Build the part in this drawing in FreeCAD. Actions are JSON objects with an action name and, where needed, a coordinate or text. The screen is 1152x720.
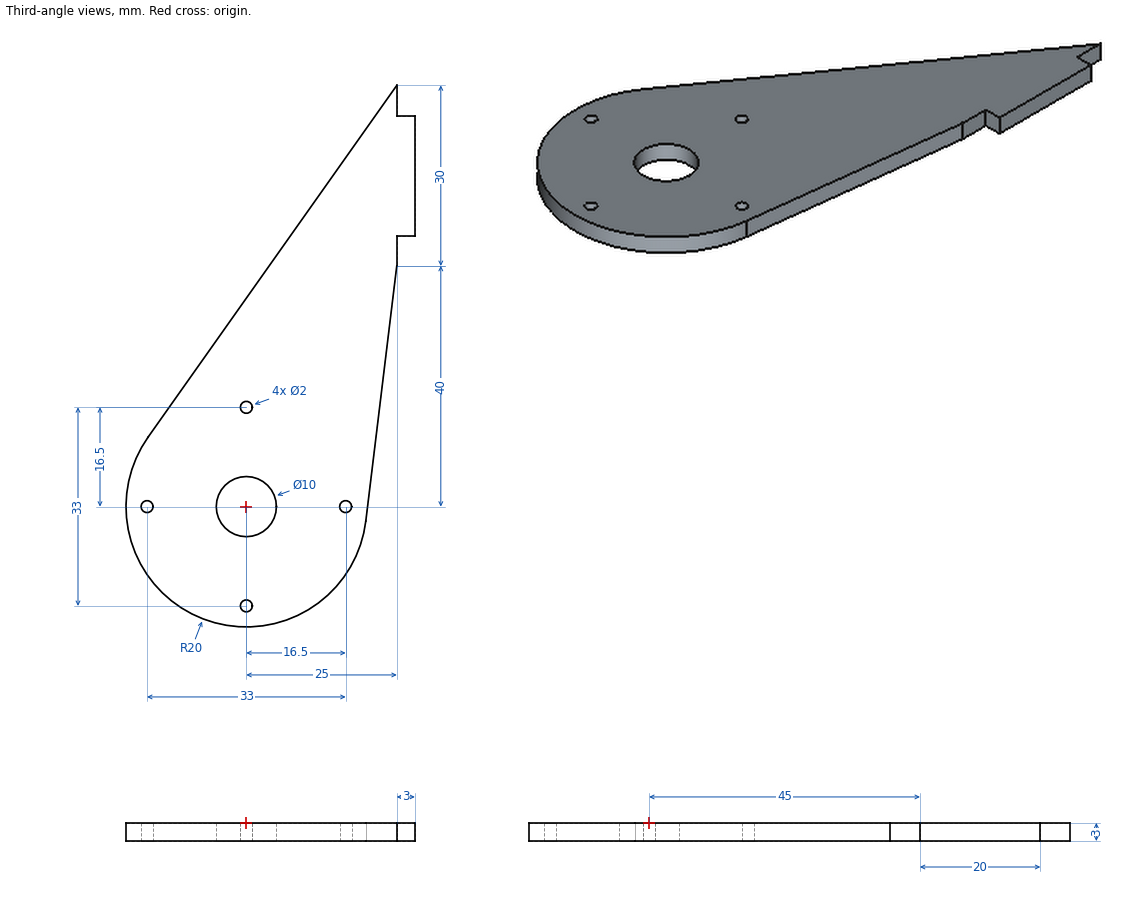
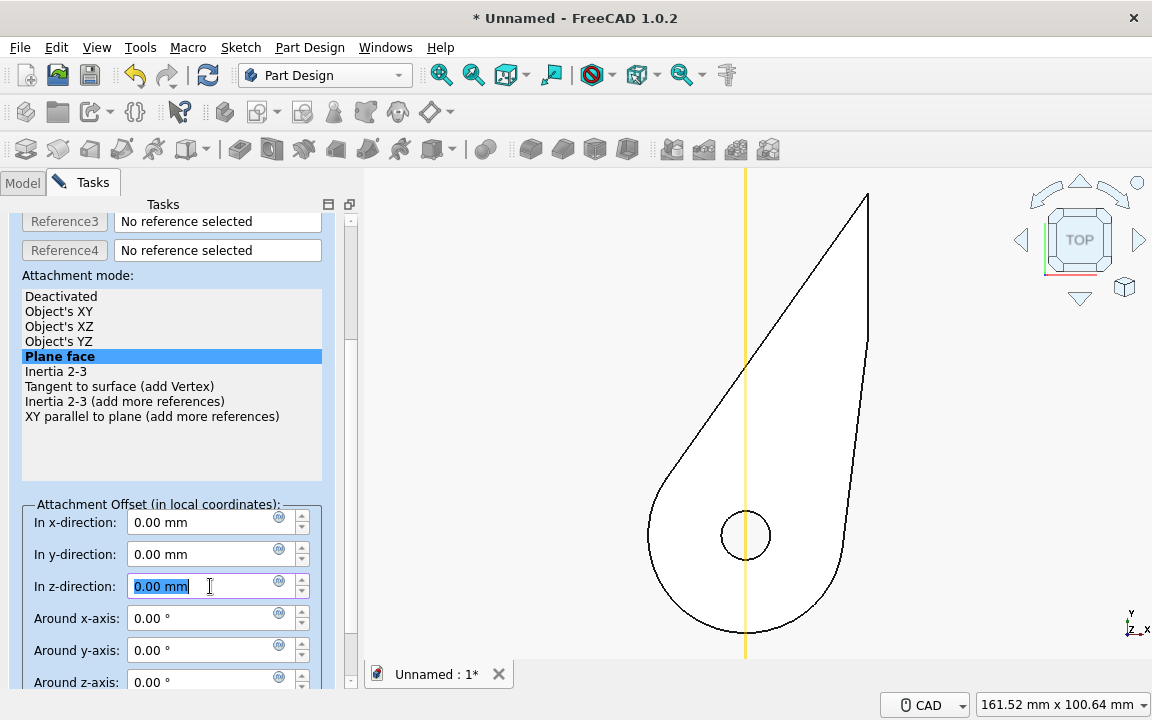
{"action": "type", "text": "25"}
{"action": "key", "text": "Tab"}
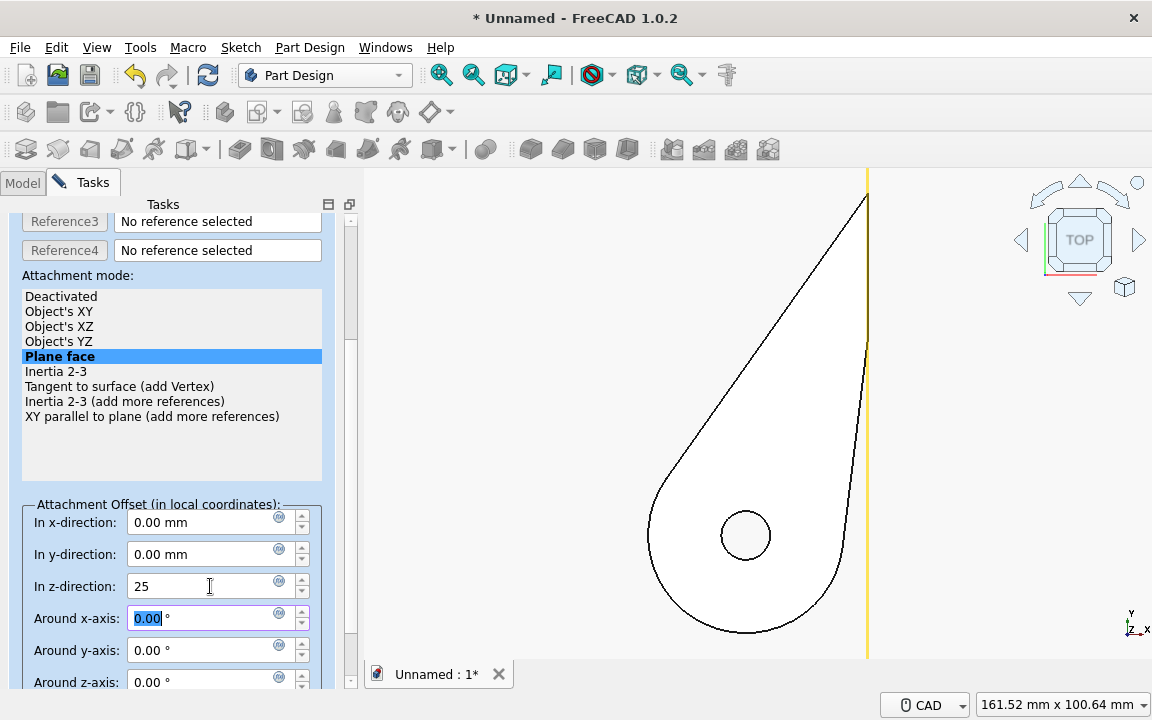
{"action": "scroll", "coordinate": [351, 451], "scroll_direction": "up", "scroll_amount": 4}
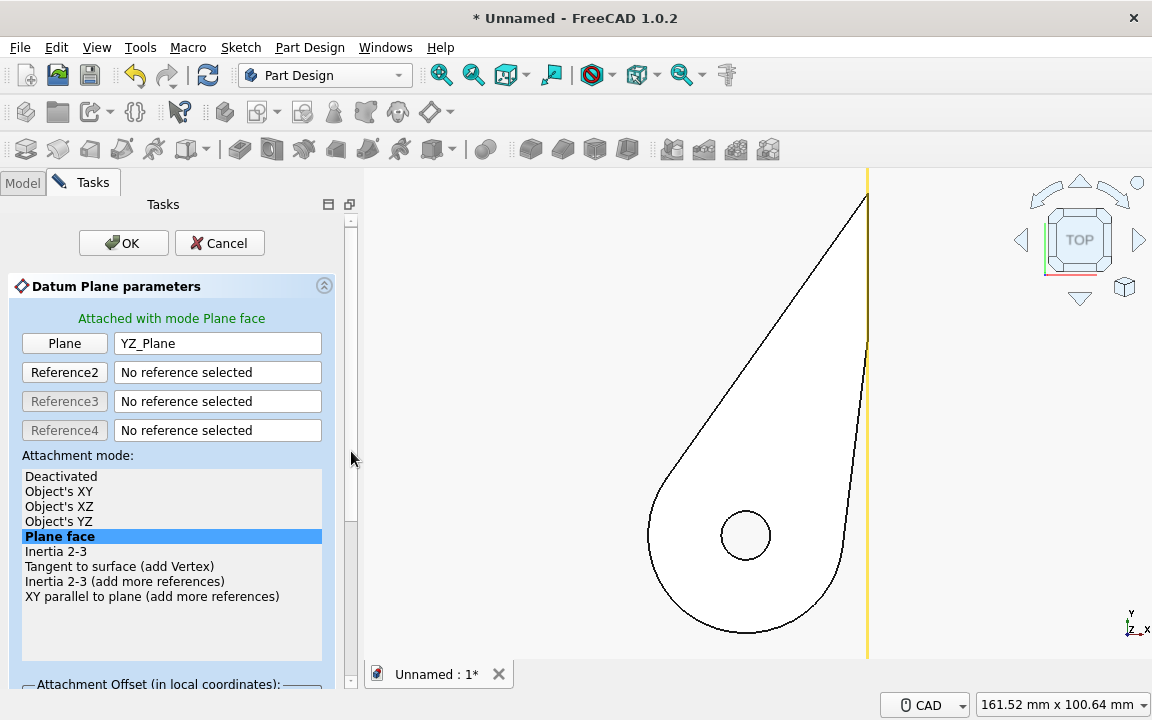
{"action": "left_click", "coordinate": [124, 243]}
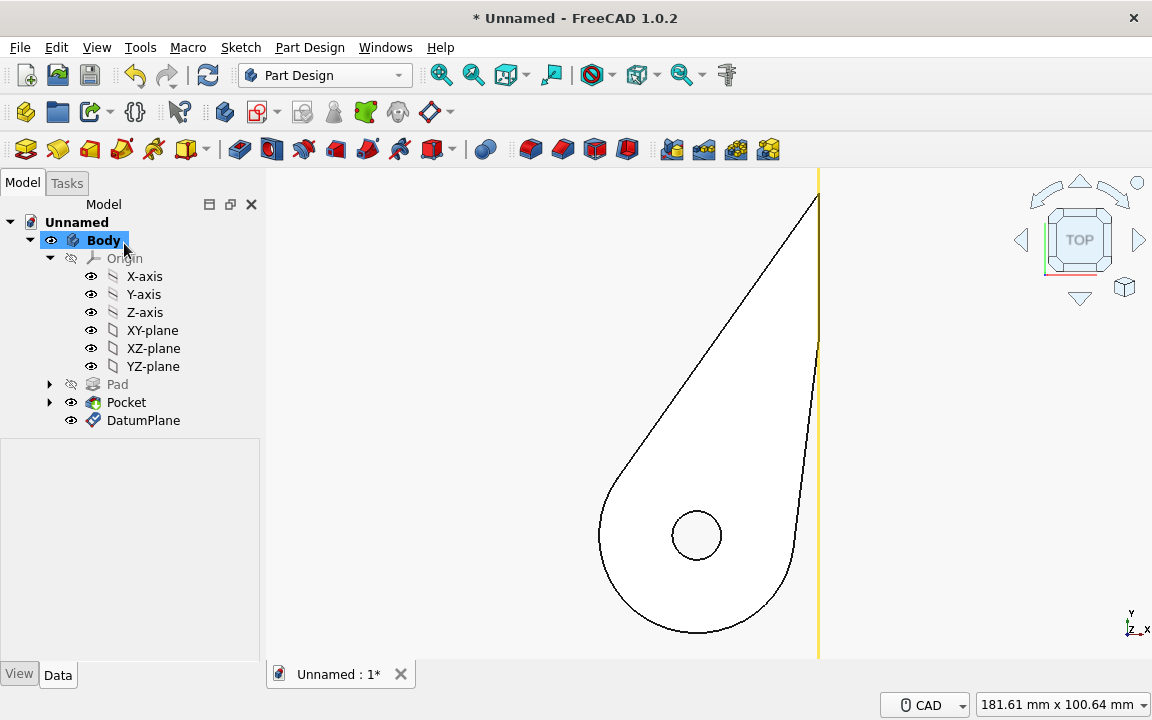
{"action": "left_click", "coordinate": [116, 420]}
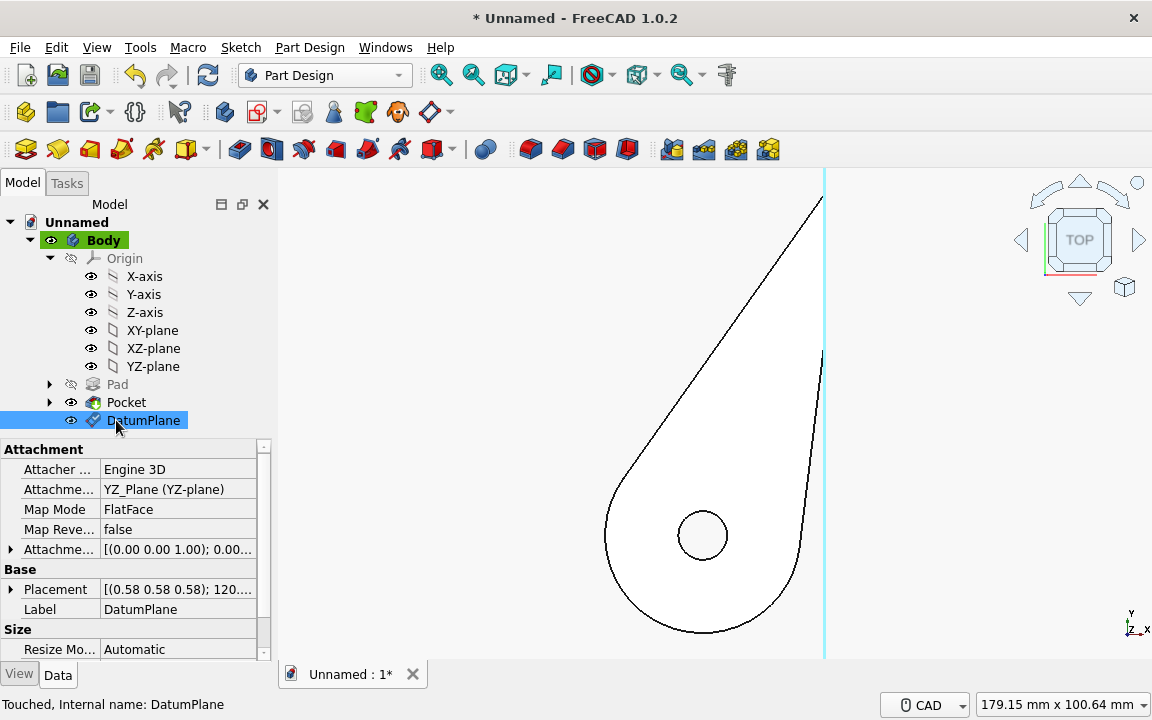
{"action": "left_click", "coordinate": [258, 112]}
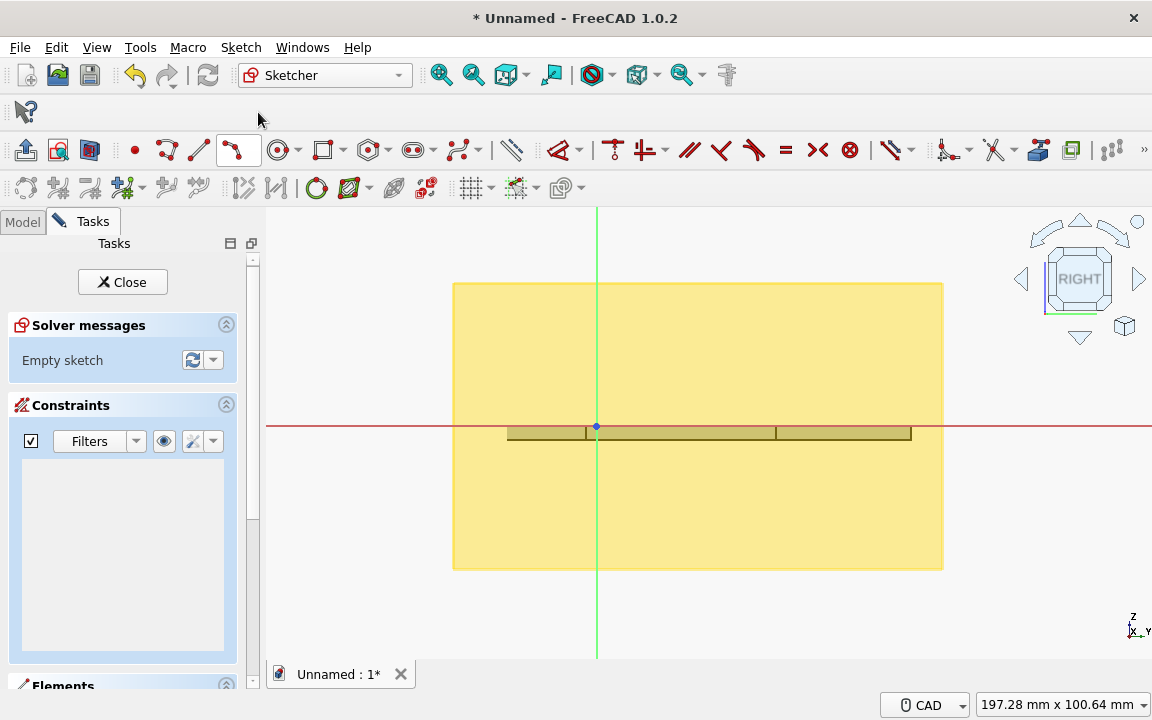
{"action": "scroll", "coordinate": [895, 433], "scroll_direction": "up", "scroll_amount": 8}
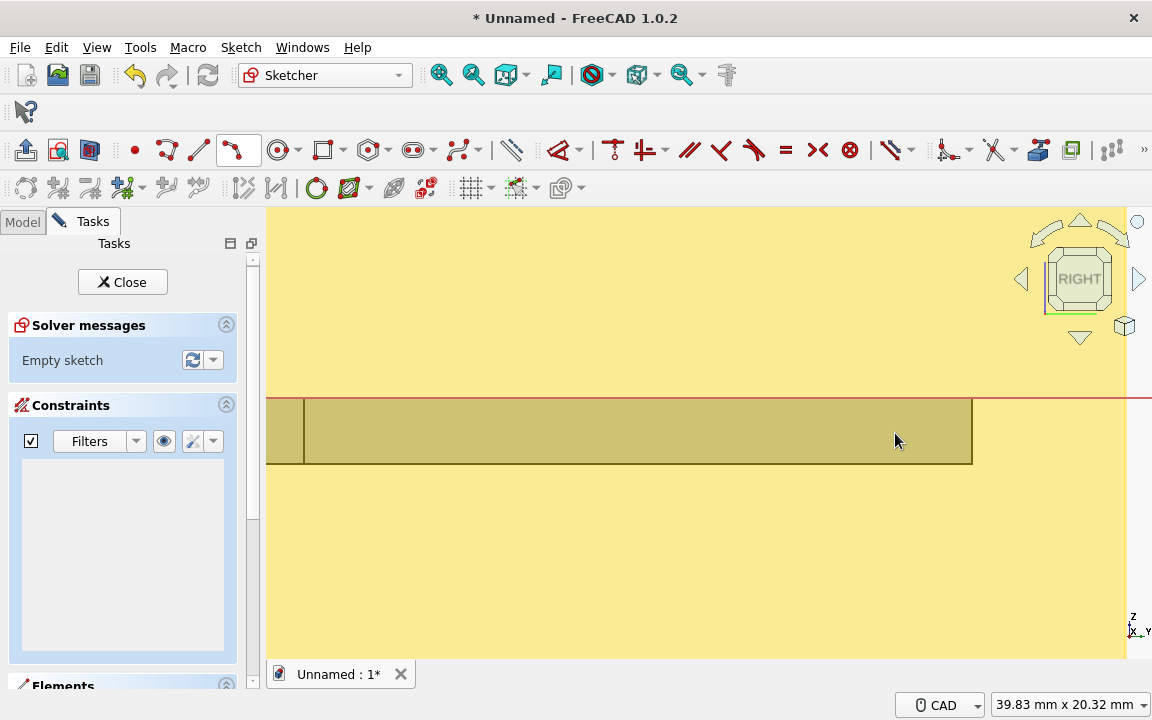
{"action": "left_click", "coordinate": [324, 150]}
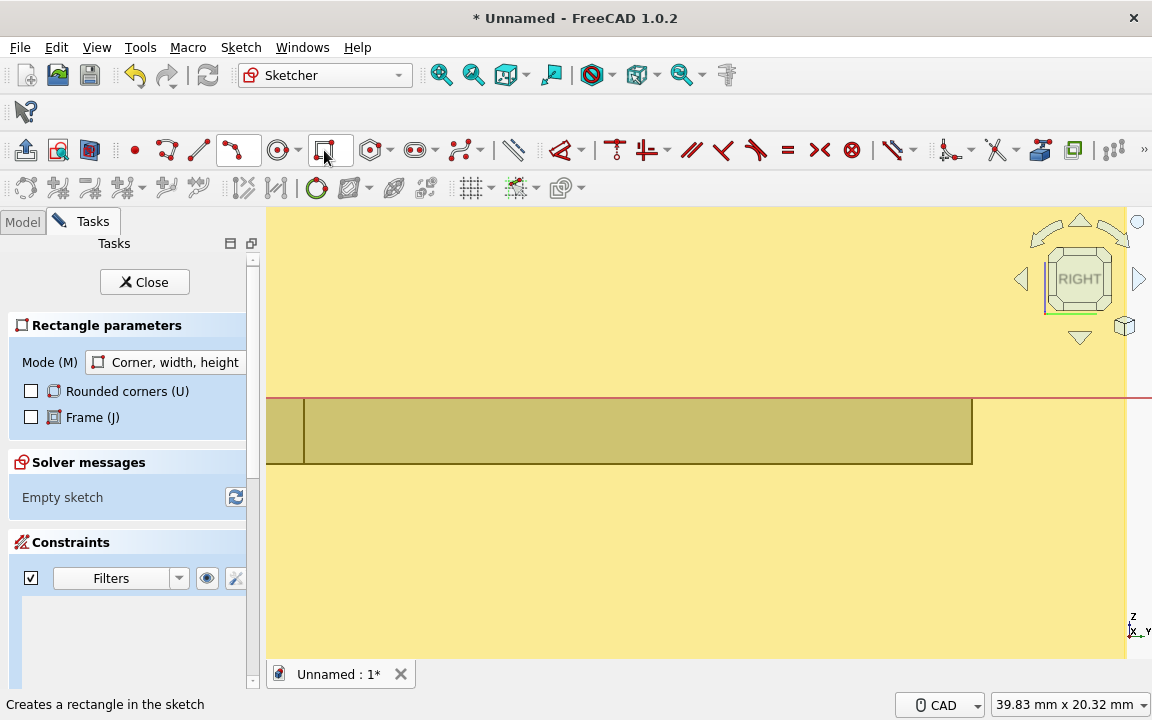
{"action": "left_click", "coordinate": [416, 398]}
{"action": "left_click", "coordinate": [861, 464]}
{"action": "key", "text": "Escape"}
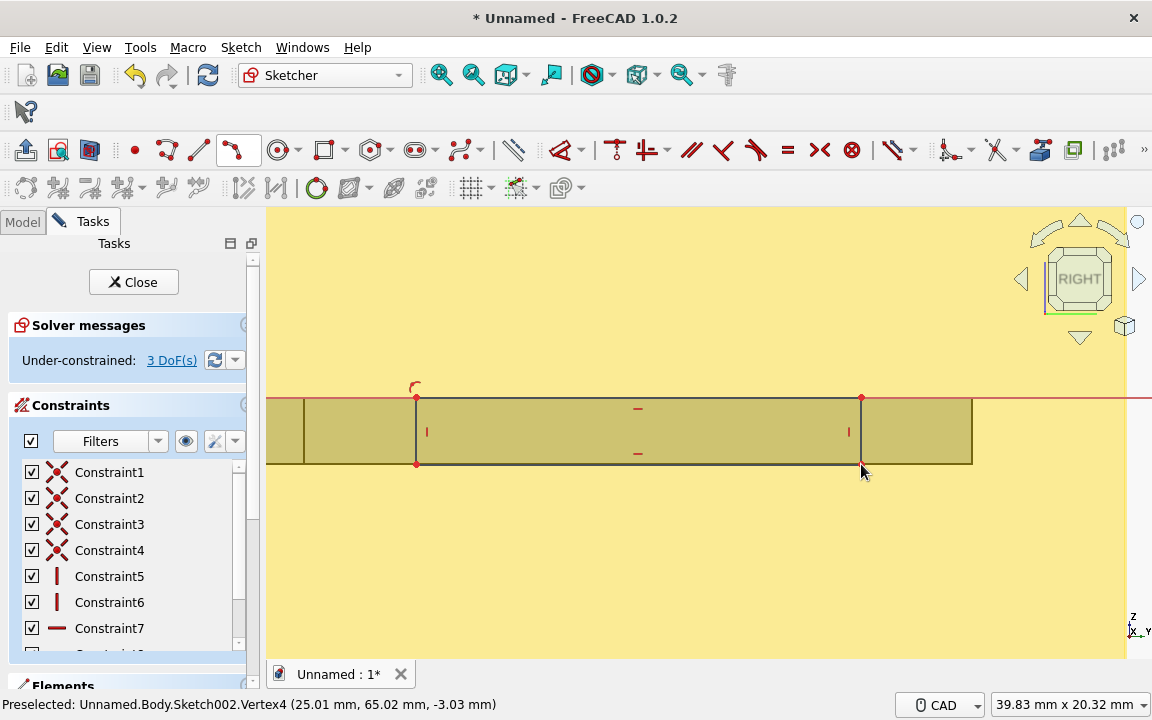
{"action": "left_click", "coordinate": [560, 150]}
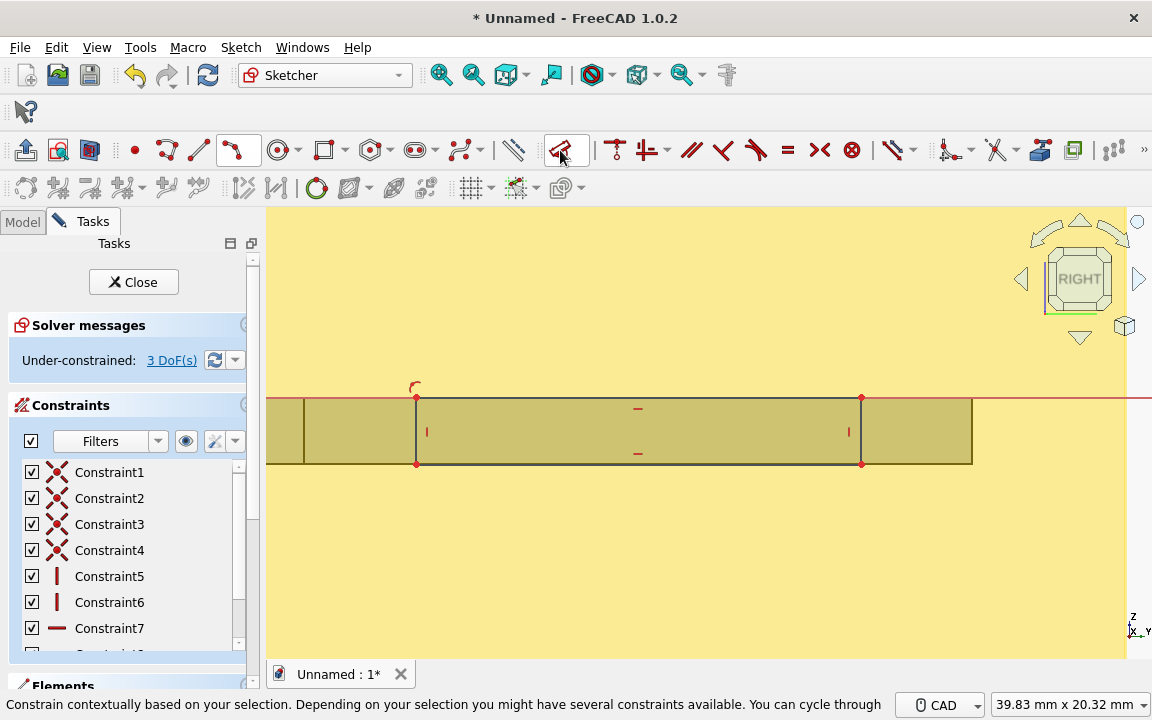
{"action": "left_click", "coordinate": [416, 418]}
{"action": "left_click", "coordinate": [382, 431]}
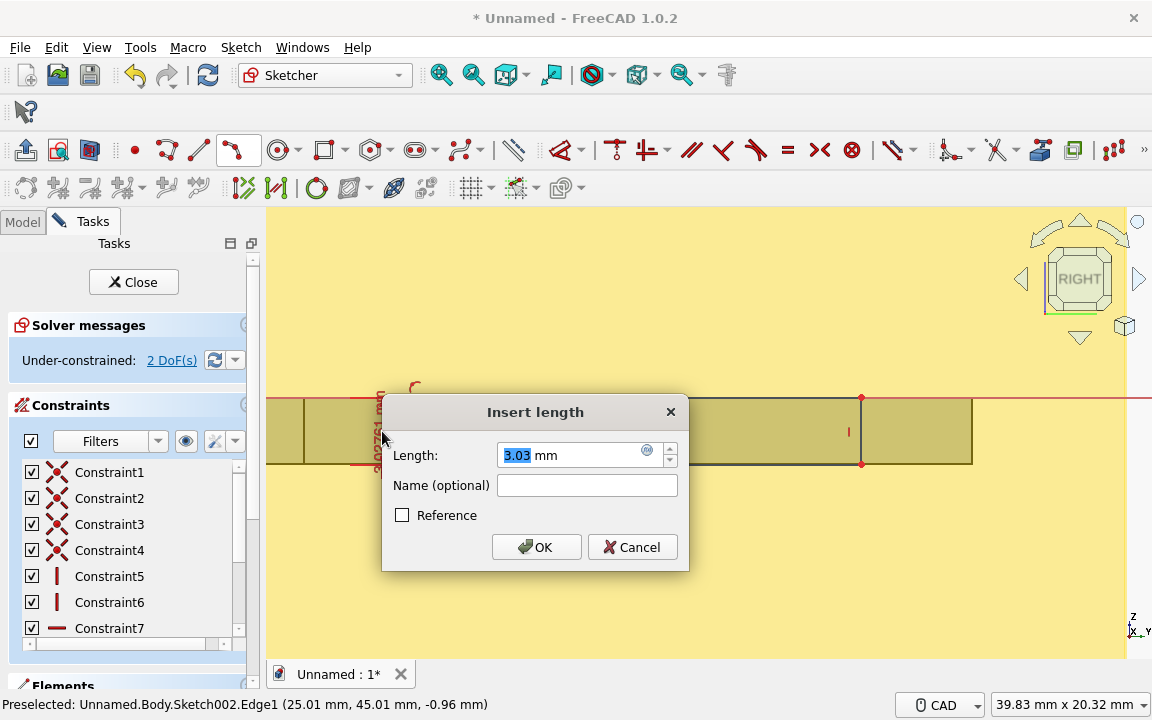
{"action": "type", "text": "3"}
{"action": "key", "text": "Return"}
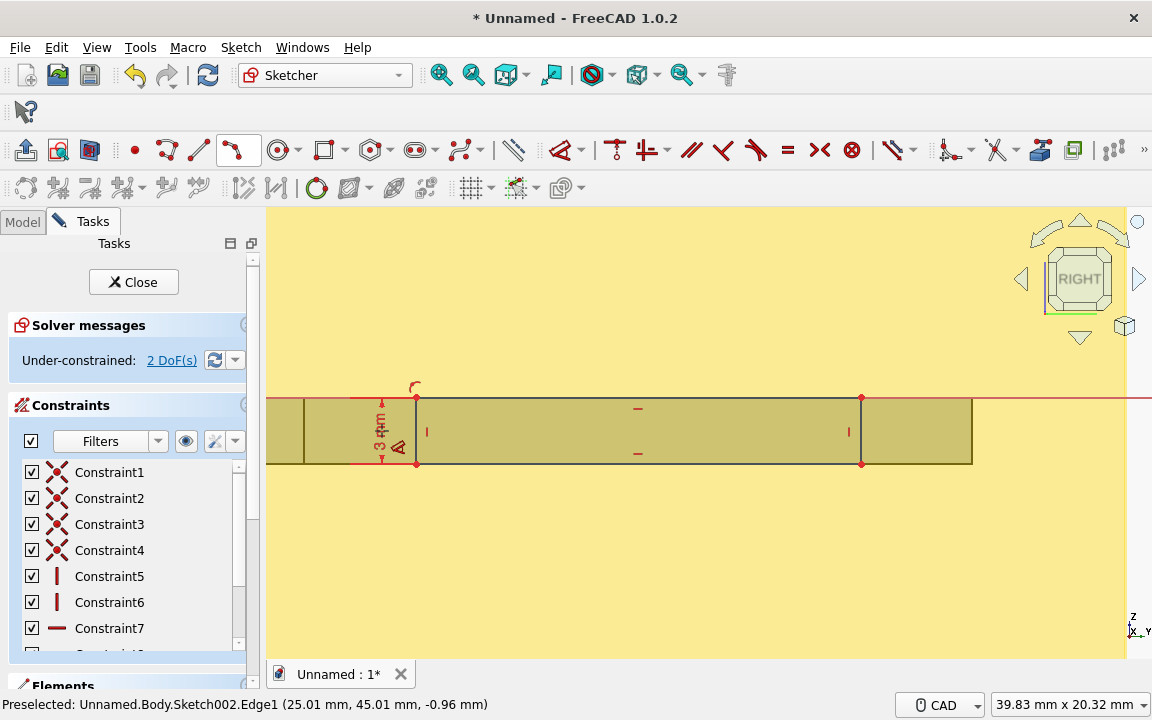
{"action": "left_click", "coordinate": [549, 464]}
{"action": "left_click", "coordinate": [638, 498]}